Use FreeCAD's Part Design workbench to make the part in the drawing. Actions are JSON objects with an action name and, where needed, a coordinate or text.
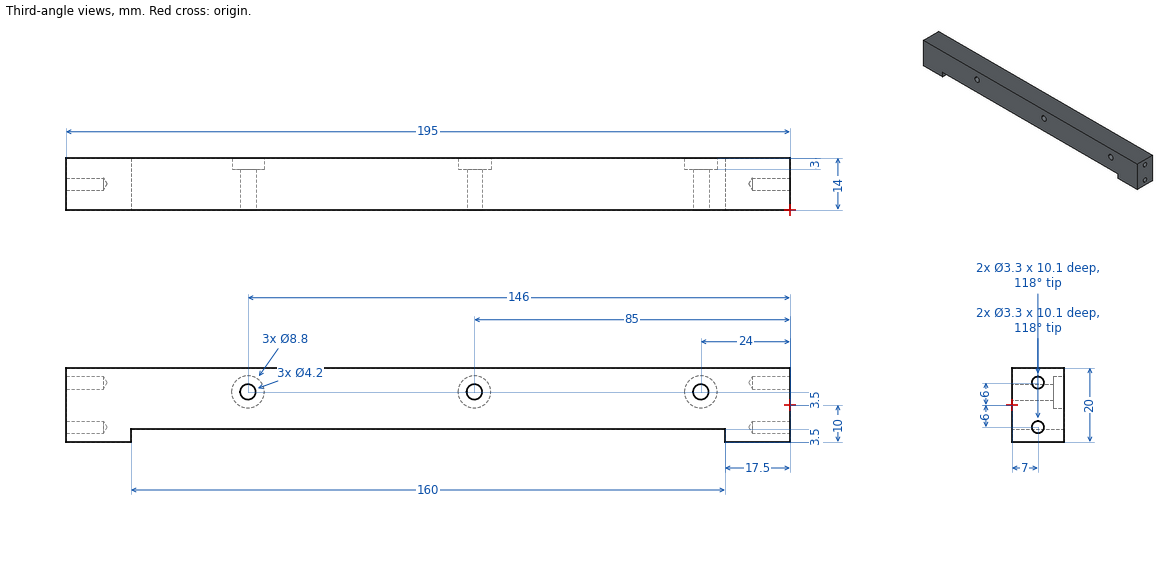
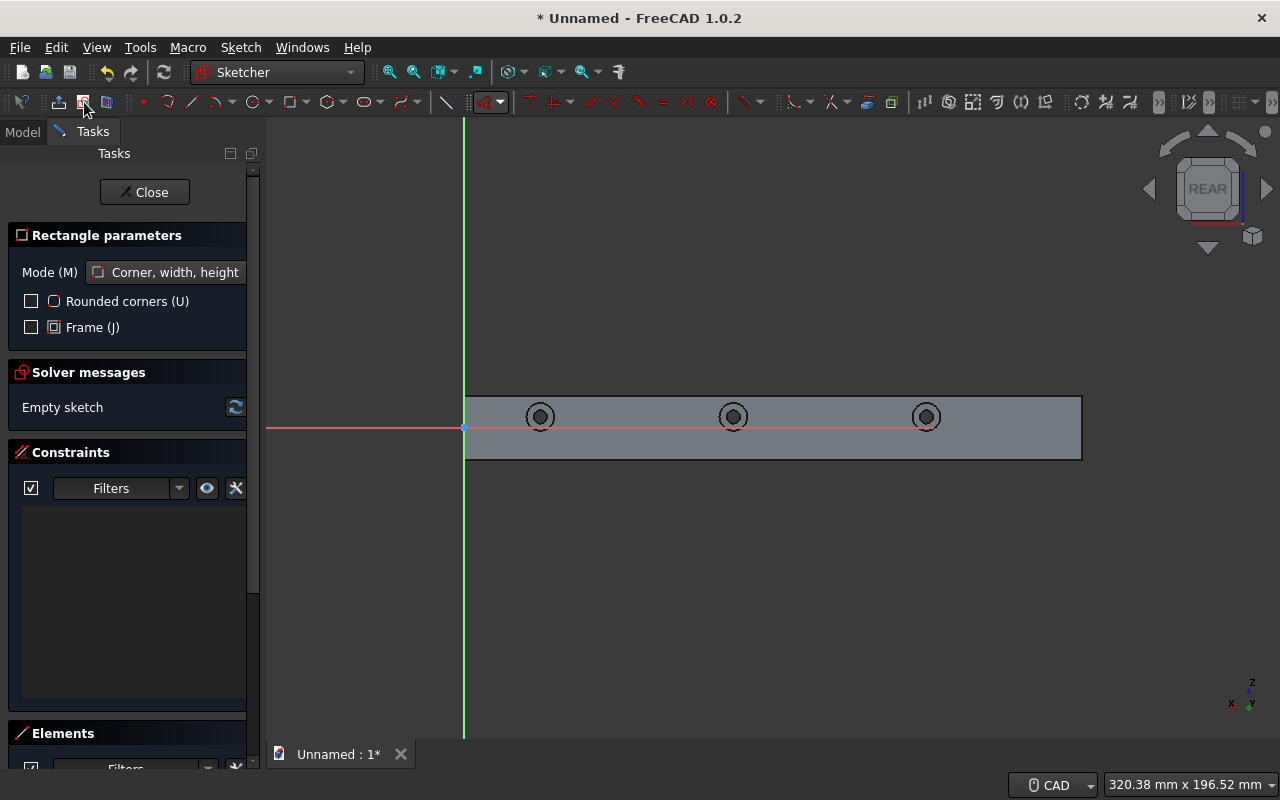
{"action": "scroll", "coordinate": [520, 449], "scroll_direction": "up", "scroll_amount": 2}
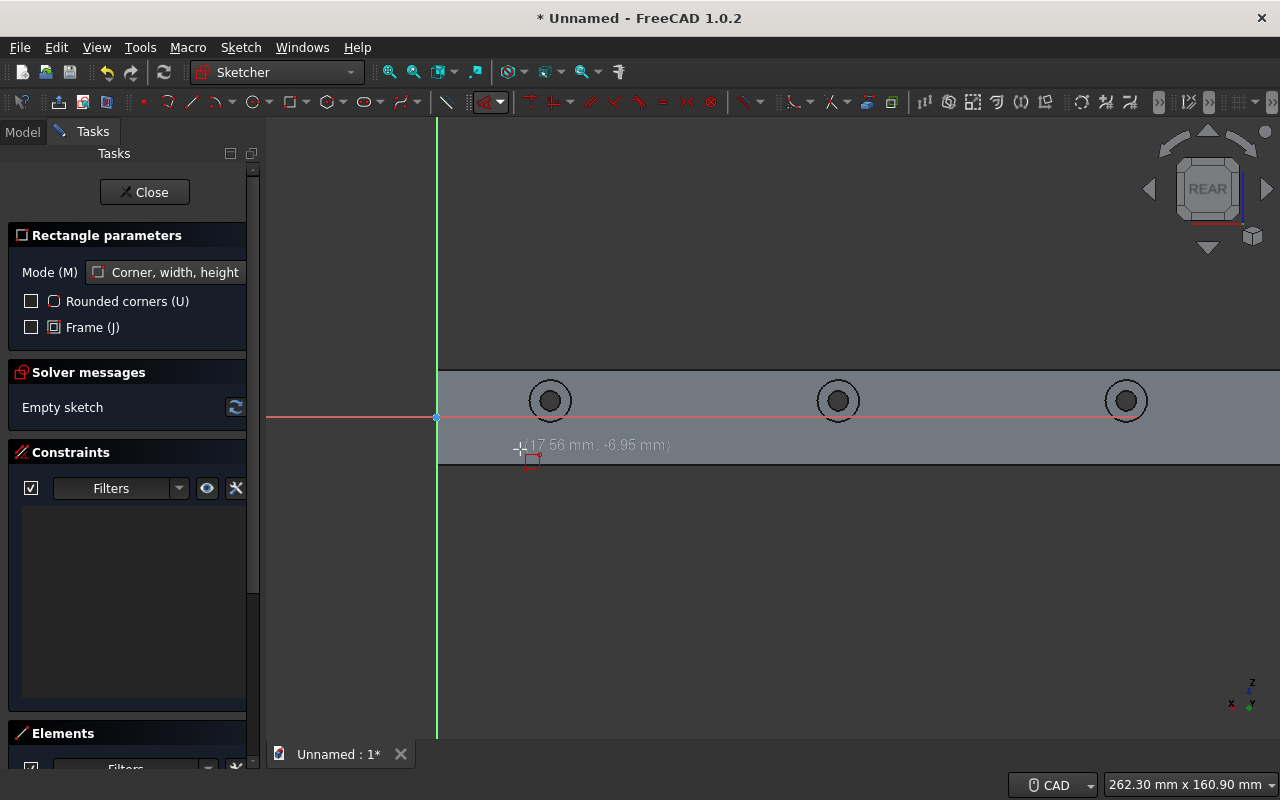
{"action": "left_click", "coordinate": [520, 448]}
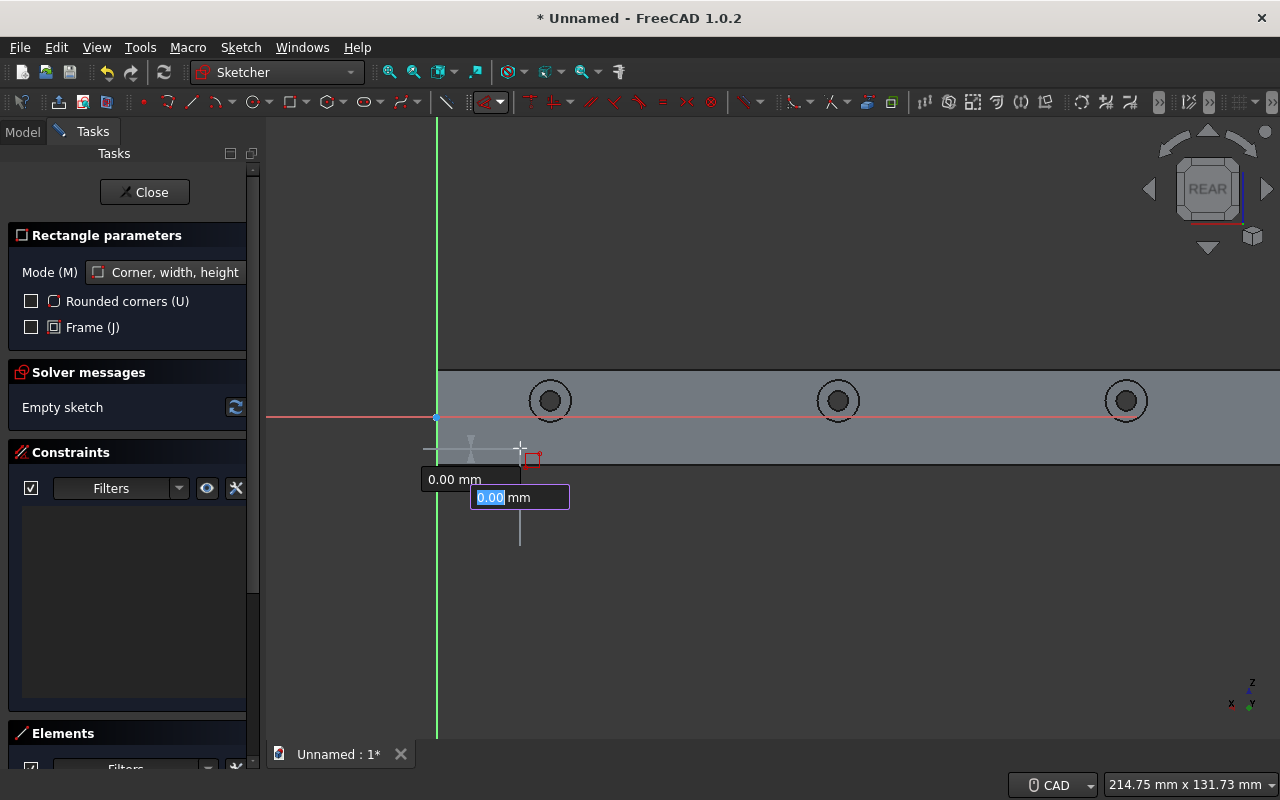
{"action": "scroll", "coordinate": [396, 402], "scroll_direction": "down", "scroll_amount": 2}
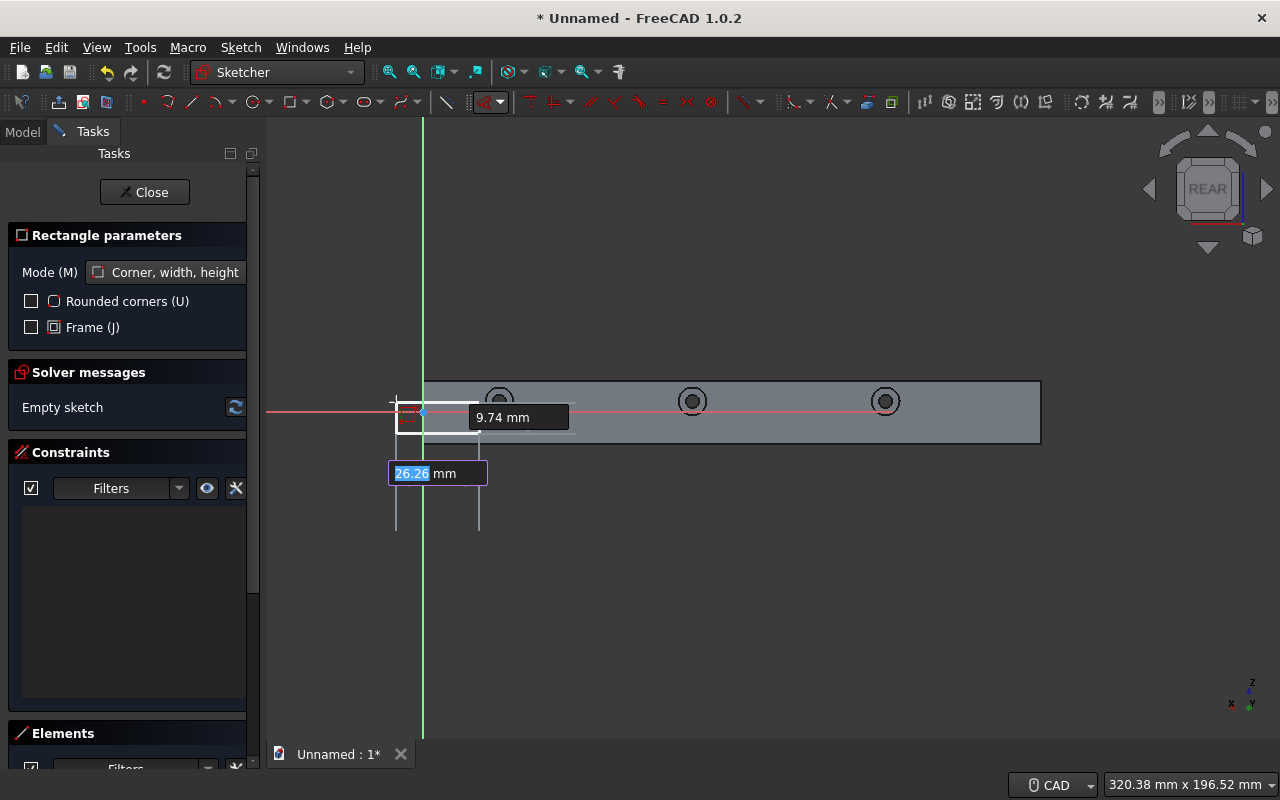
{"action": "left_click", "coordinate": [985, 444]}
{"action": "key", "text": "Escape"}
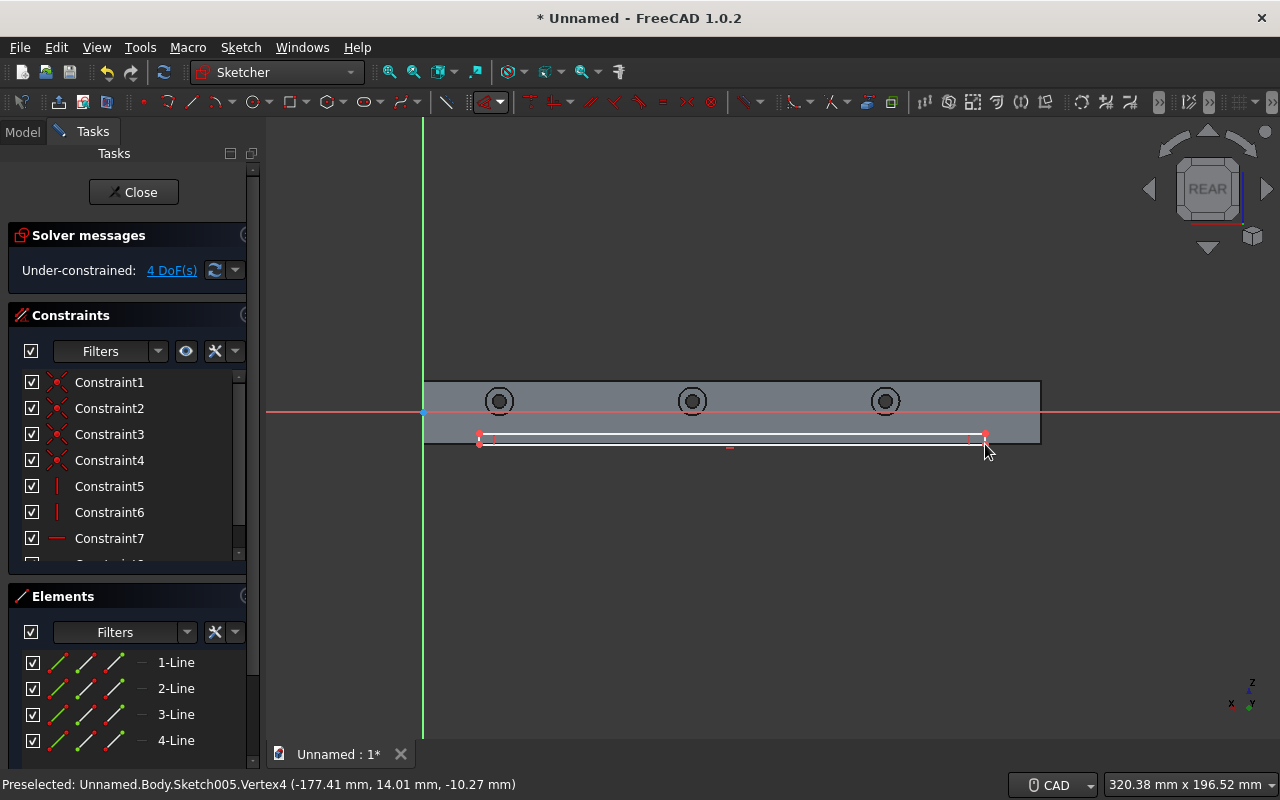
{"action": "scroll", "coordinate": [479, 439], "scroll_direction": "up", "scroll_amount": 7}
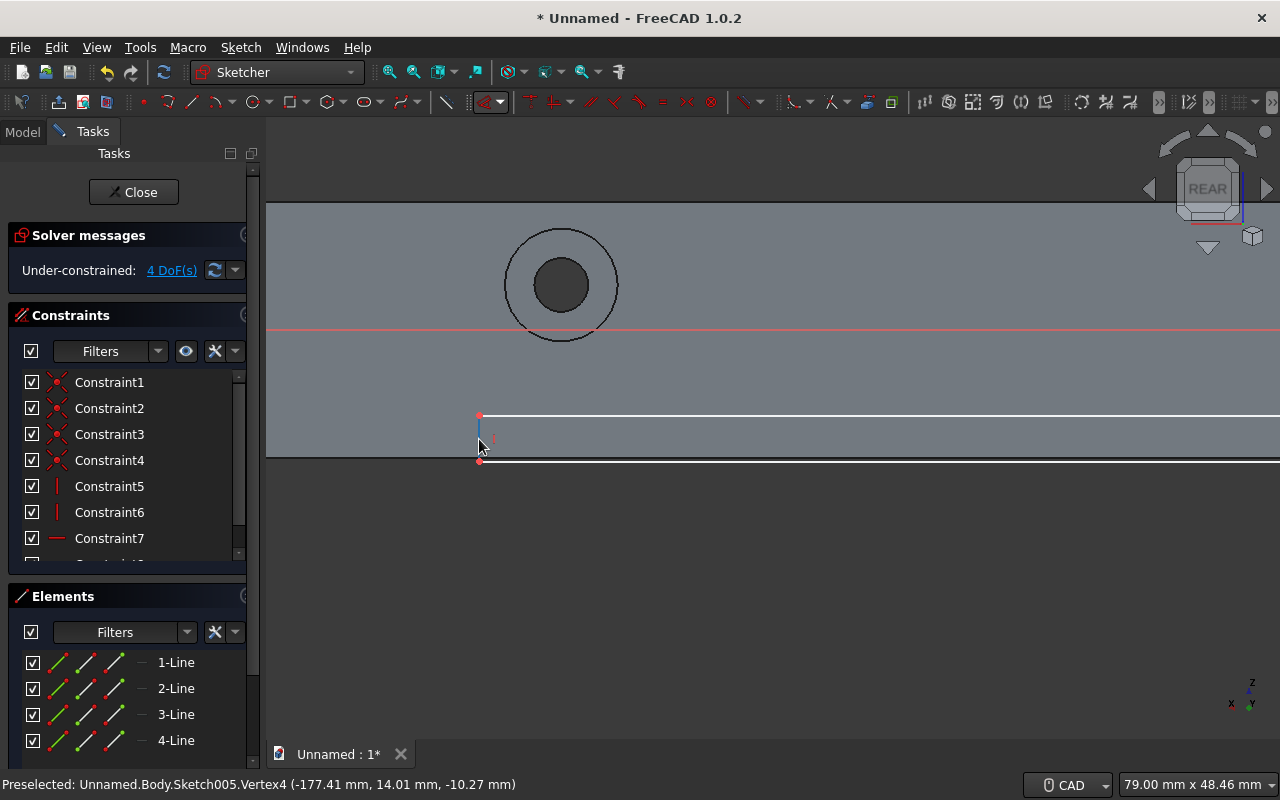
{"action": "left_click", "coordinate": [479, 439]}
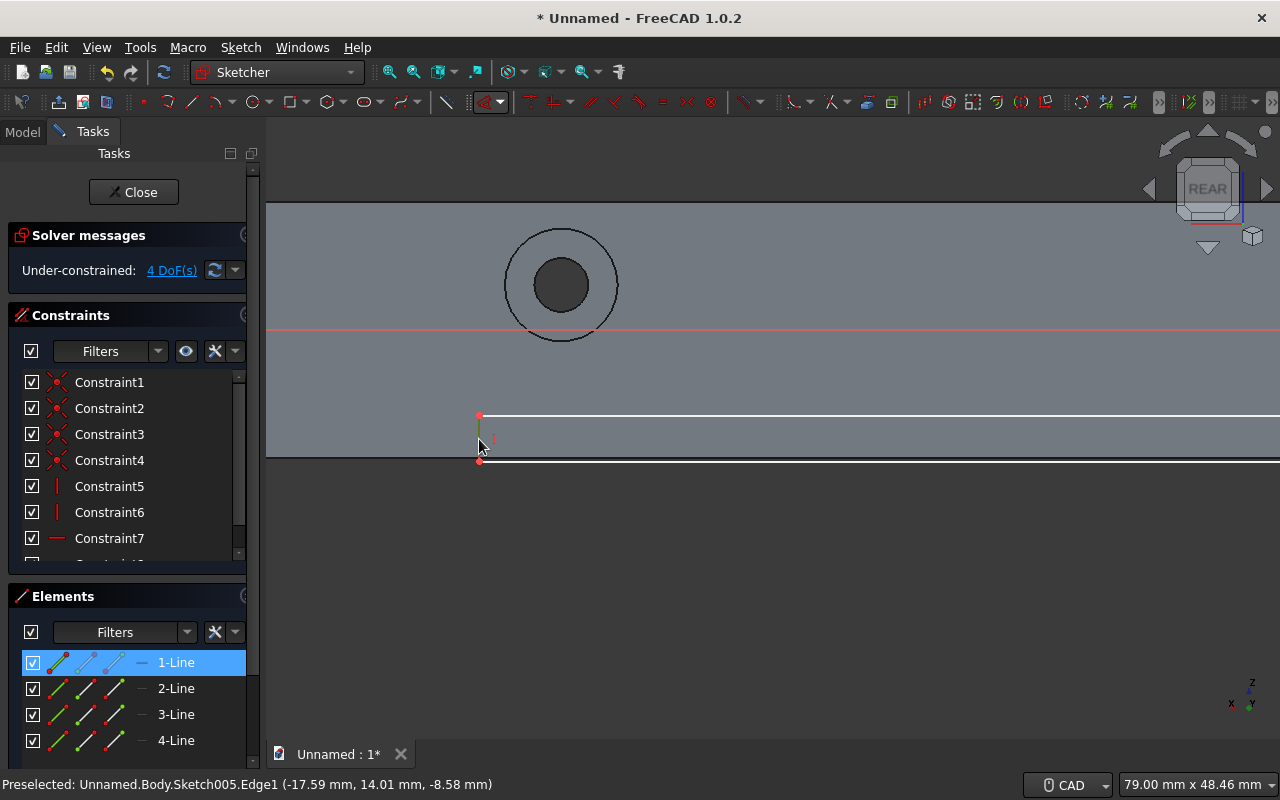
{"action": "key", "text": "i"}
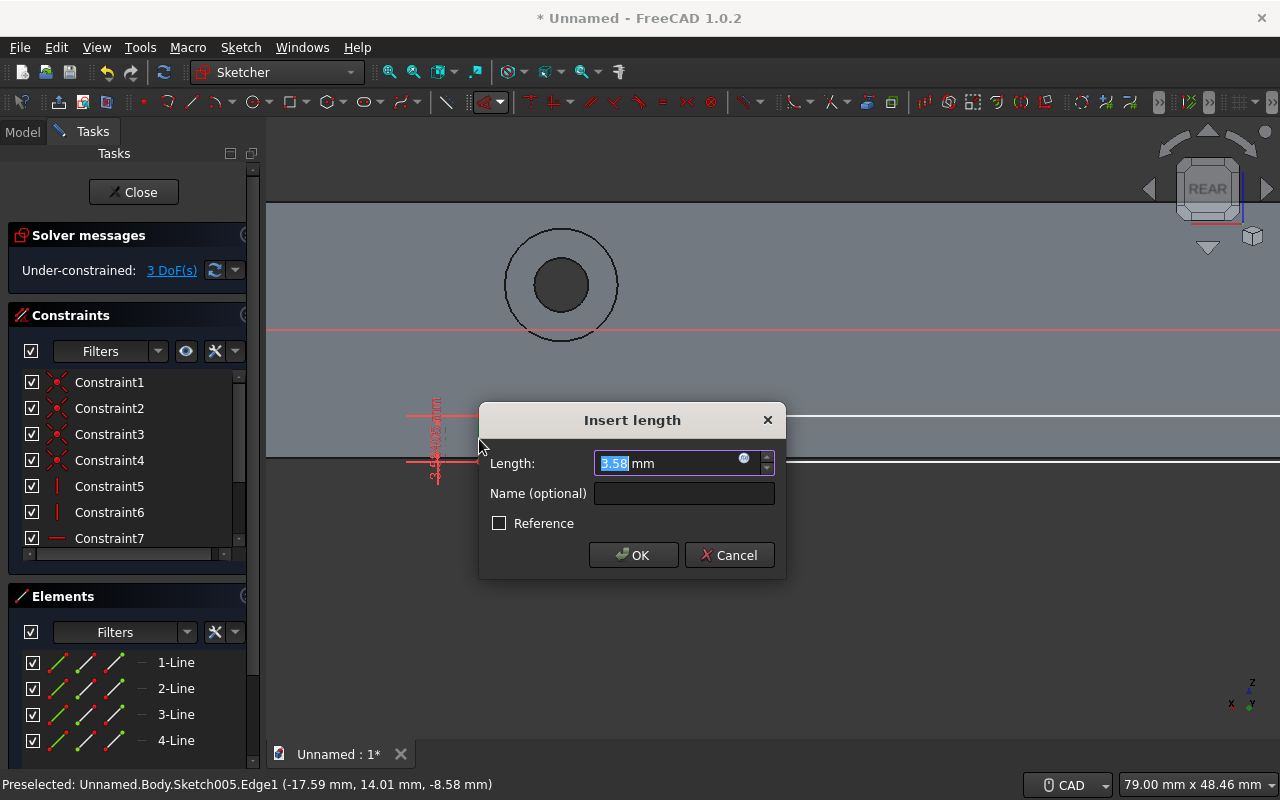
{"action": "type", "text": "3.5"}
{"action": "key", "text": "Return"}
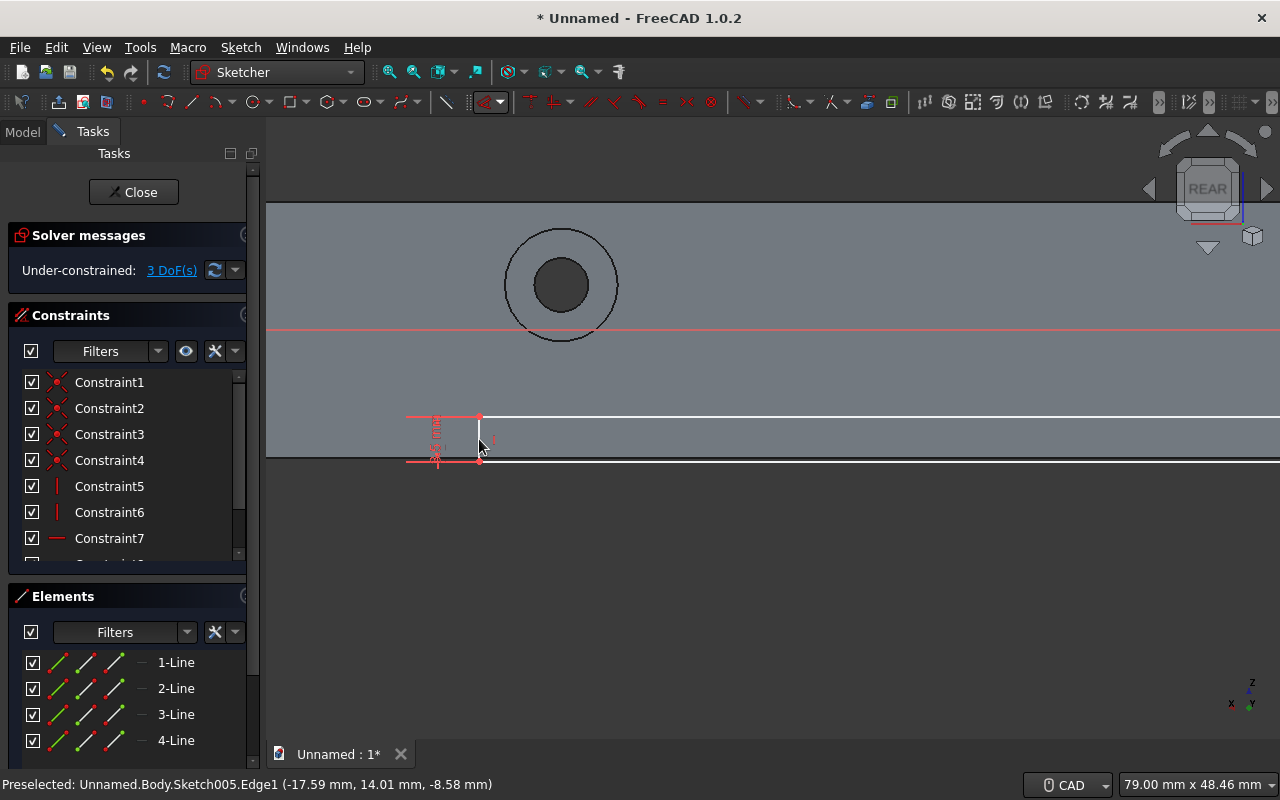
{"action": "scroll", "coordinate": [479, 439], "scroll_direction": "down", "scroll_amount": 7}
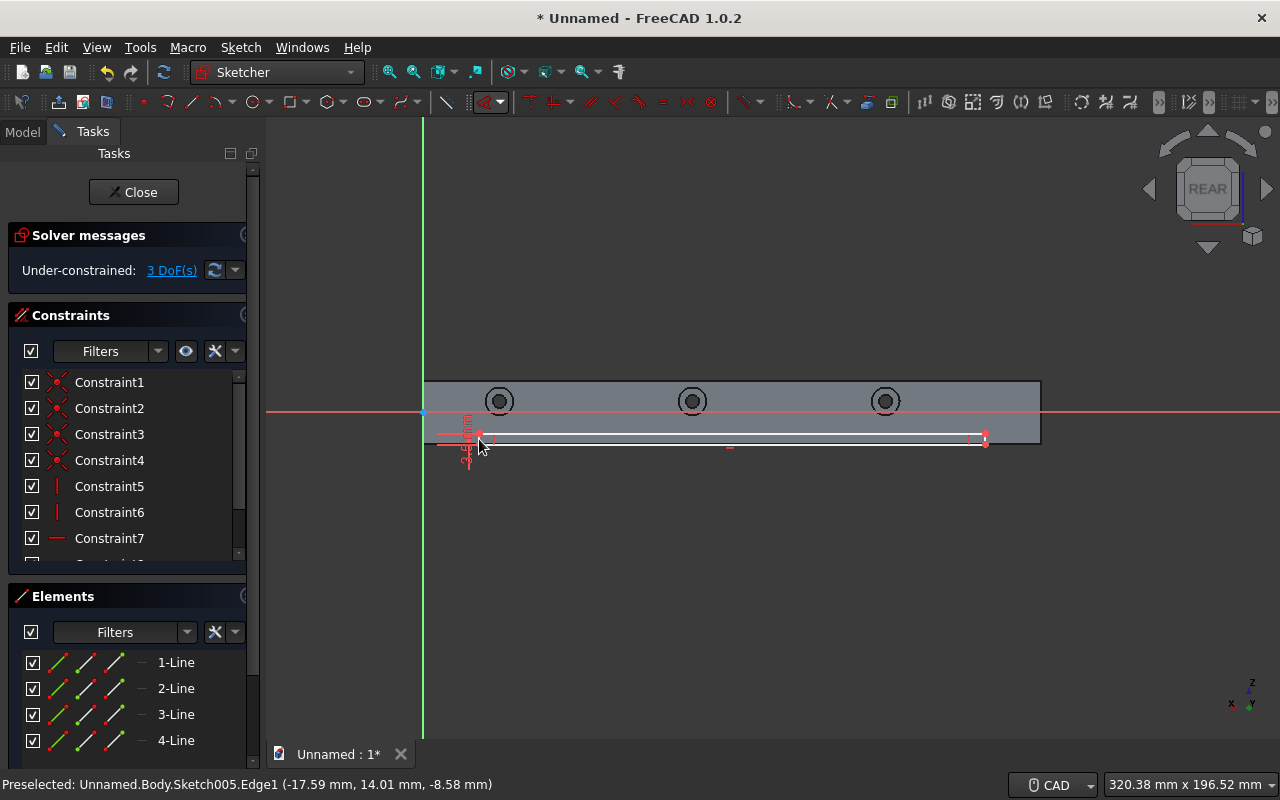
{"action": "scroll", "coordinate": [631, 445], "scroll_direction": "up", "scroll_amount": 2}